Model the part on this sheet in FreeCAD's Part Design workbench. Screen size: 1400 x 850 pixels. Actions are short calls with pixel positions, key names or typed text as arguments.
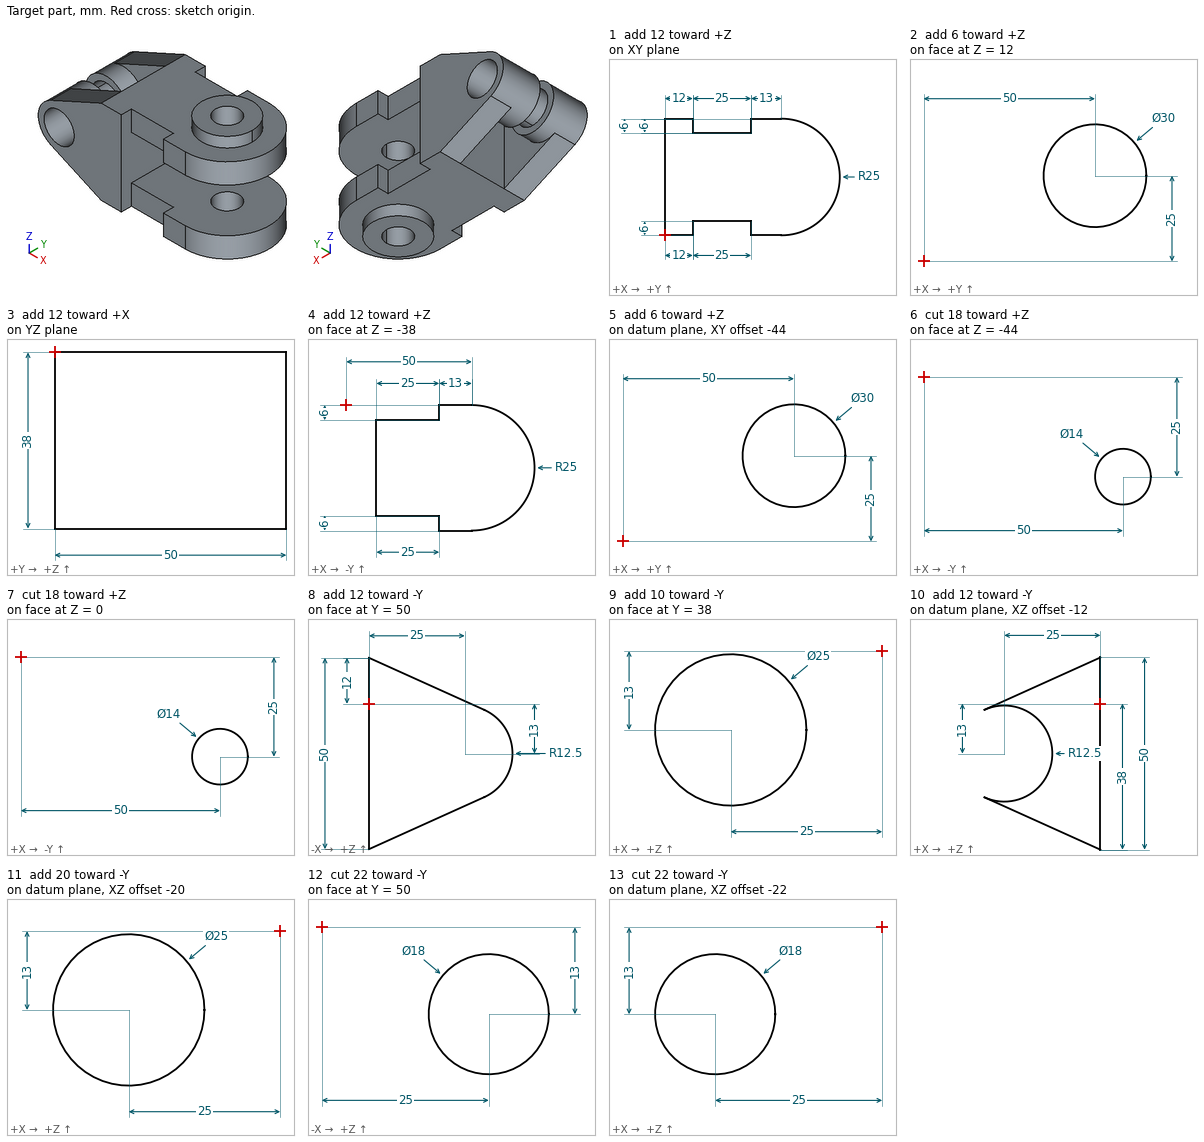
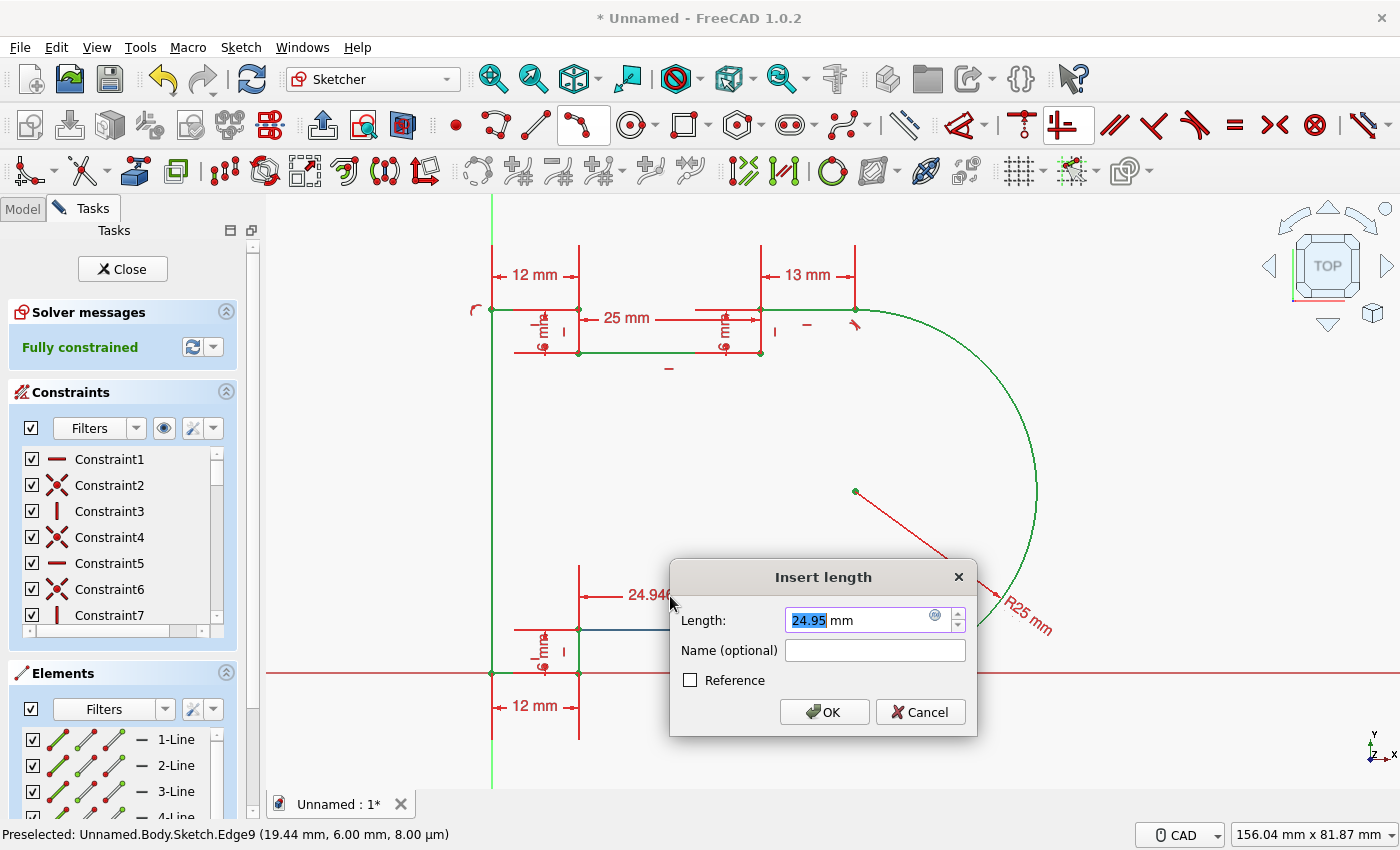
text(25)
key(Return)
key(Escape)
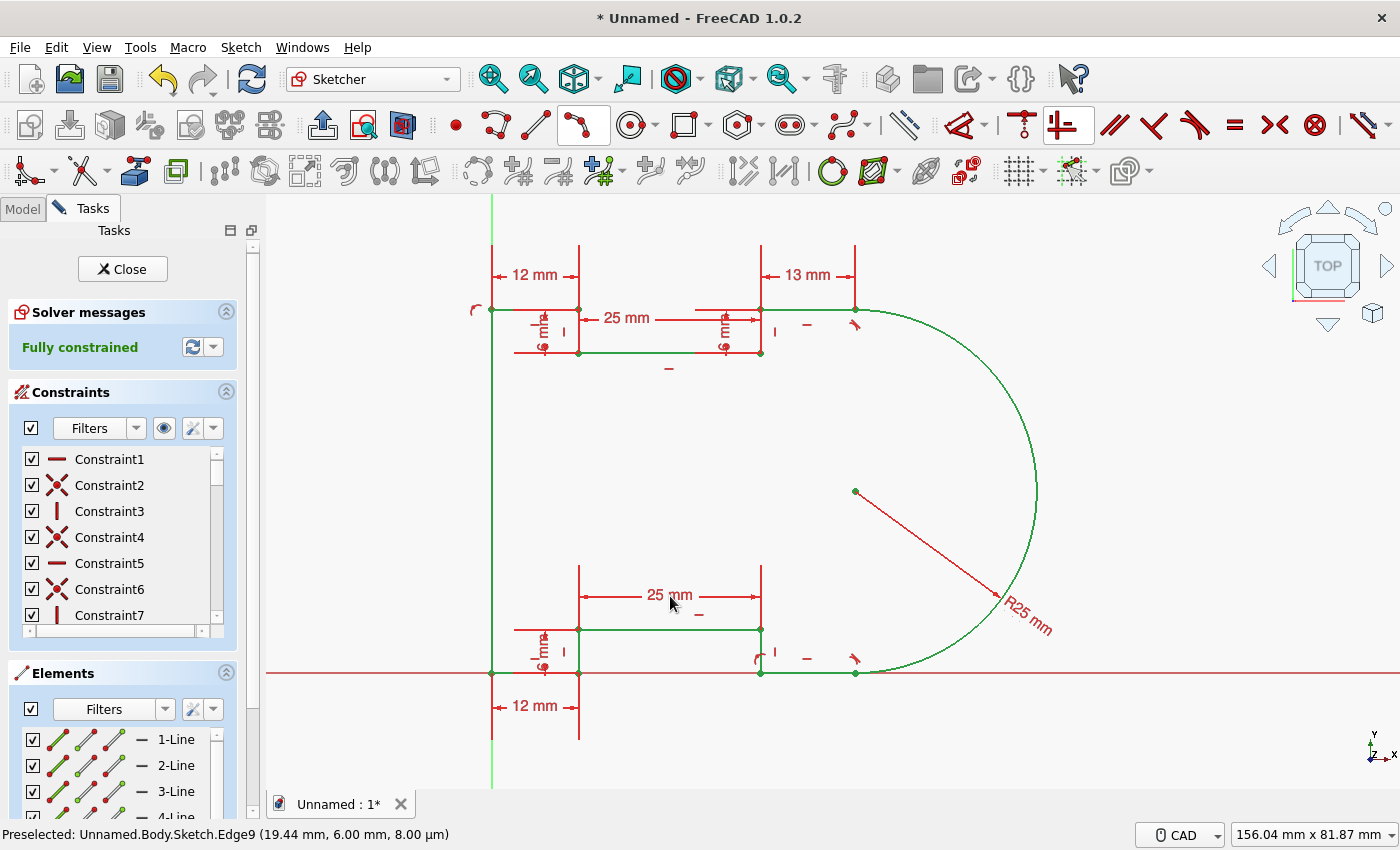
click(123, 269)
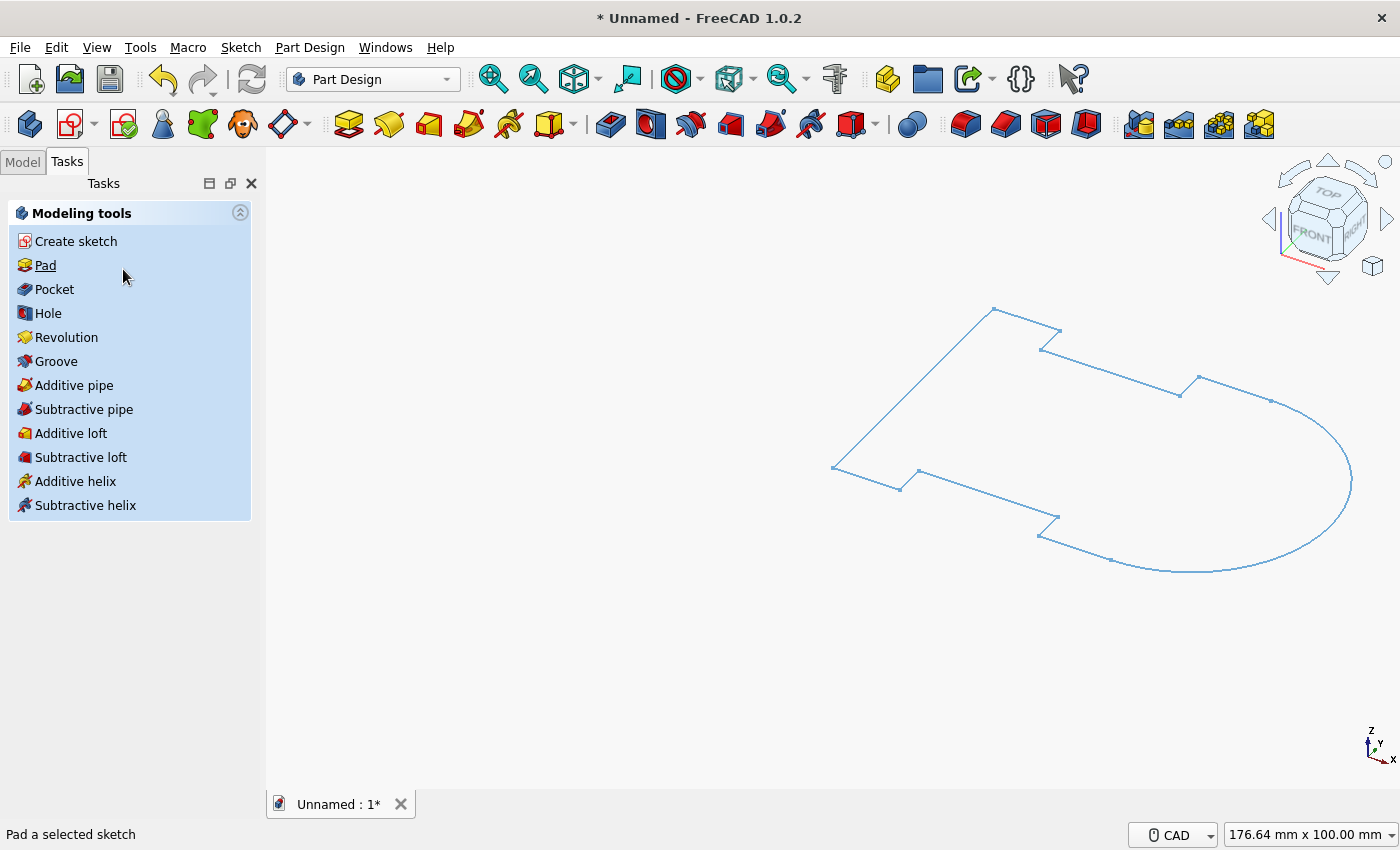
click(350, 124)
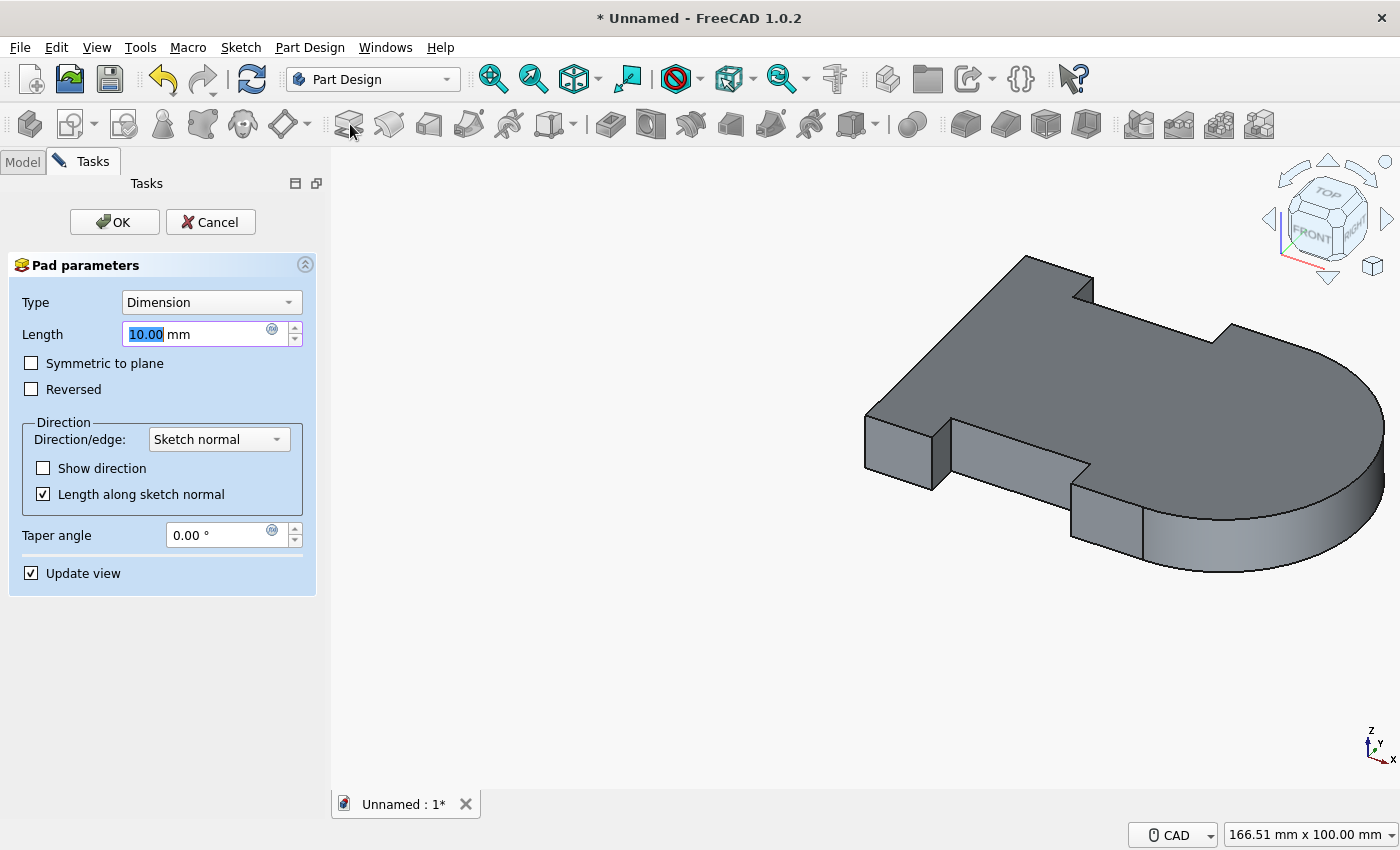
text(12)
key(Tab)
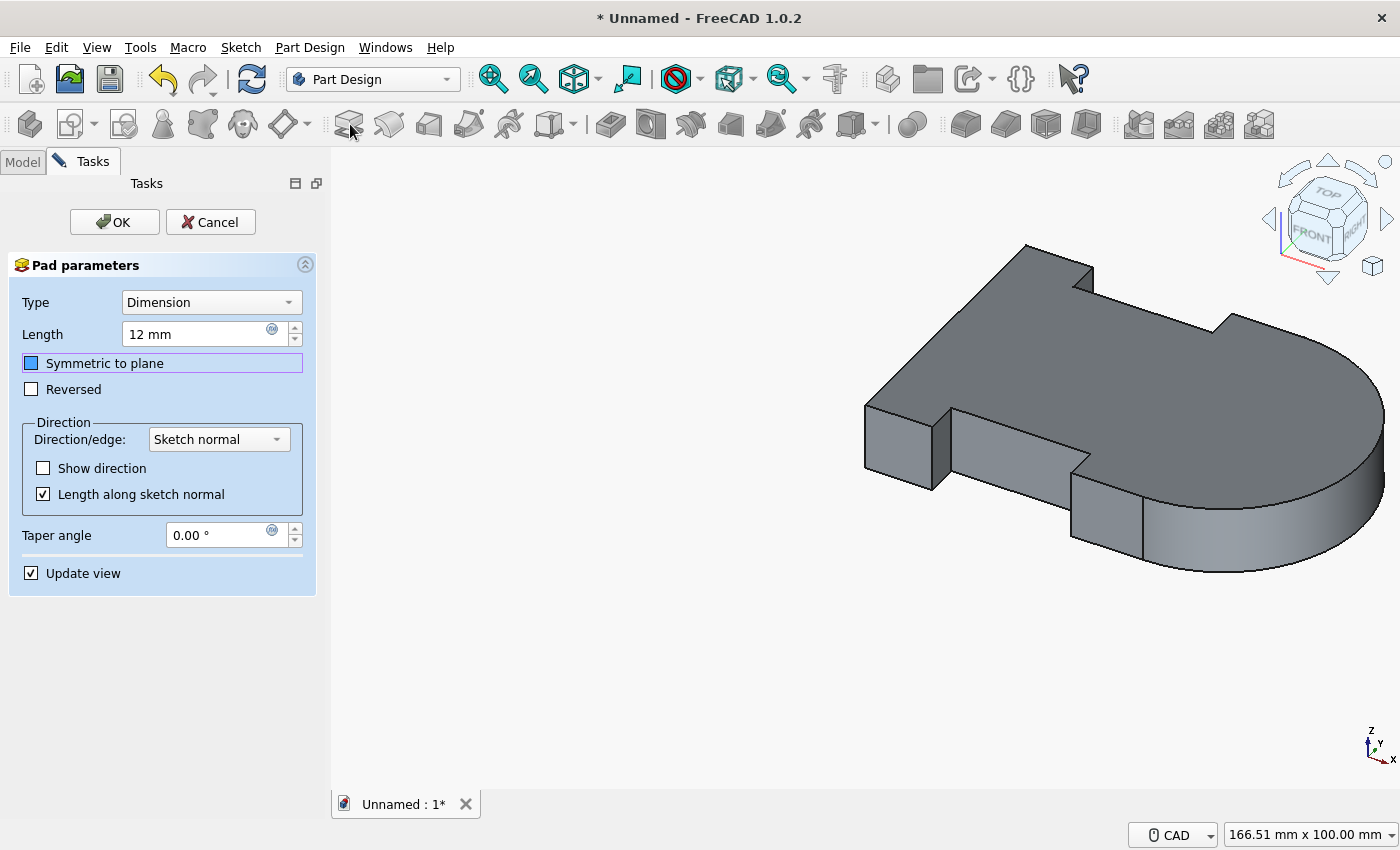
click(115, 222)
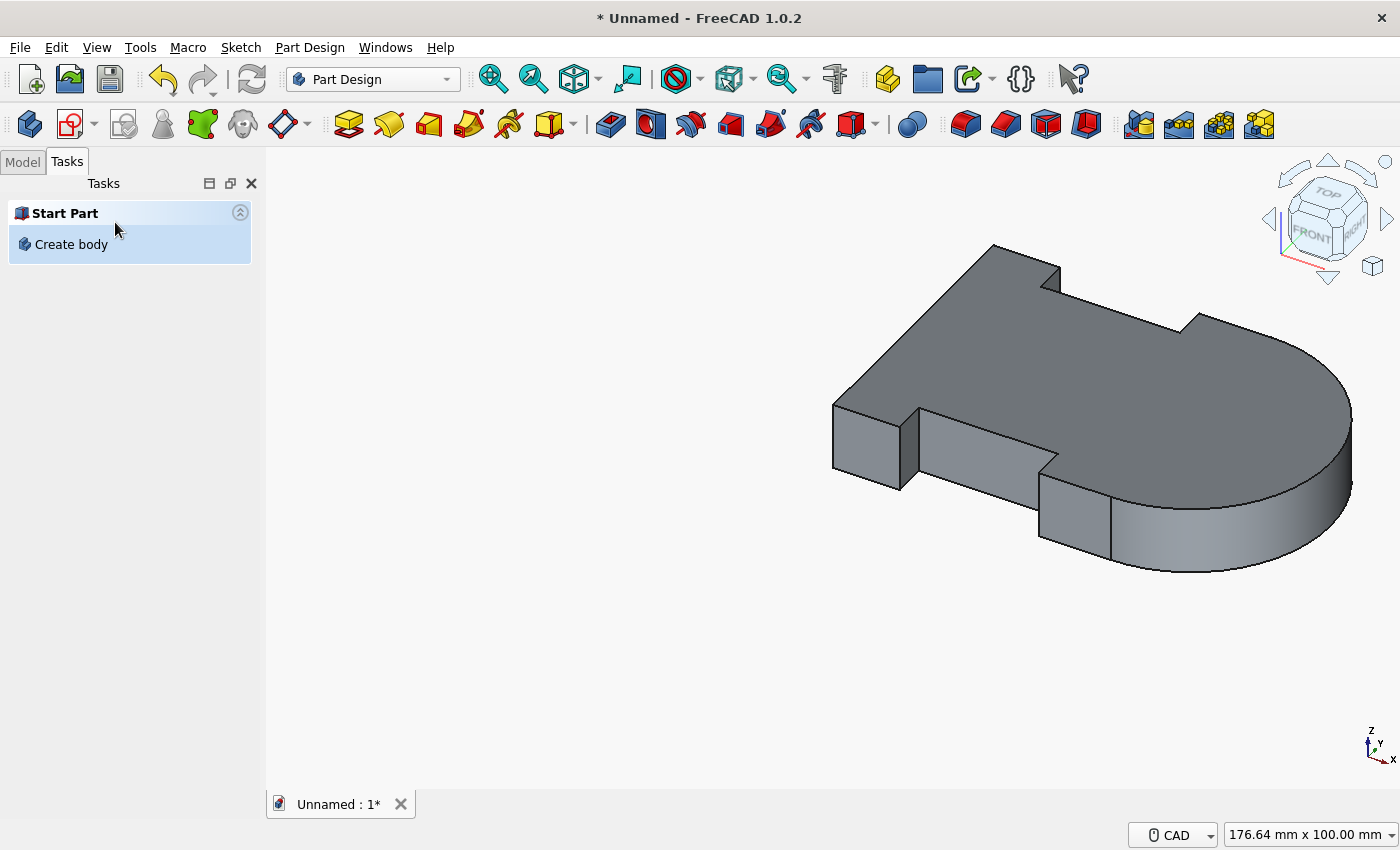
click(494, 80)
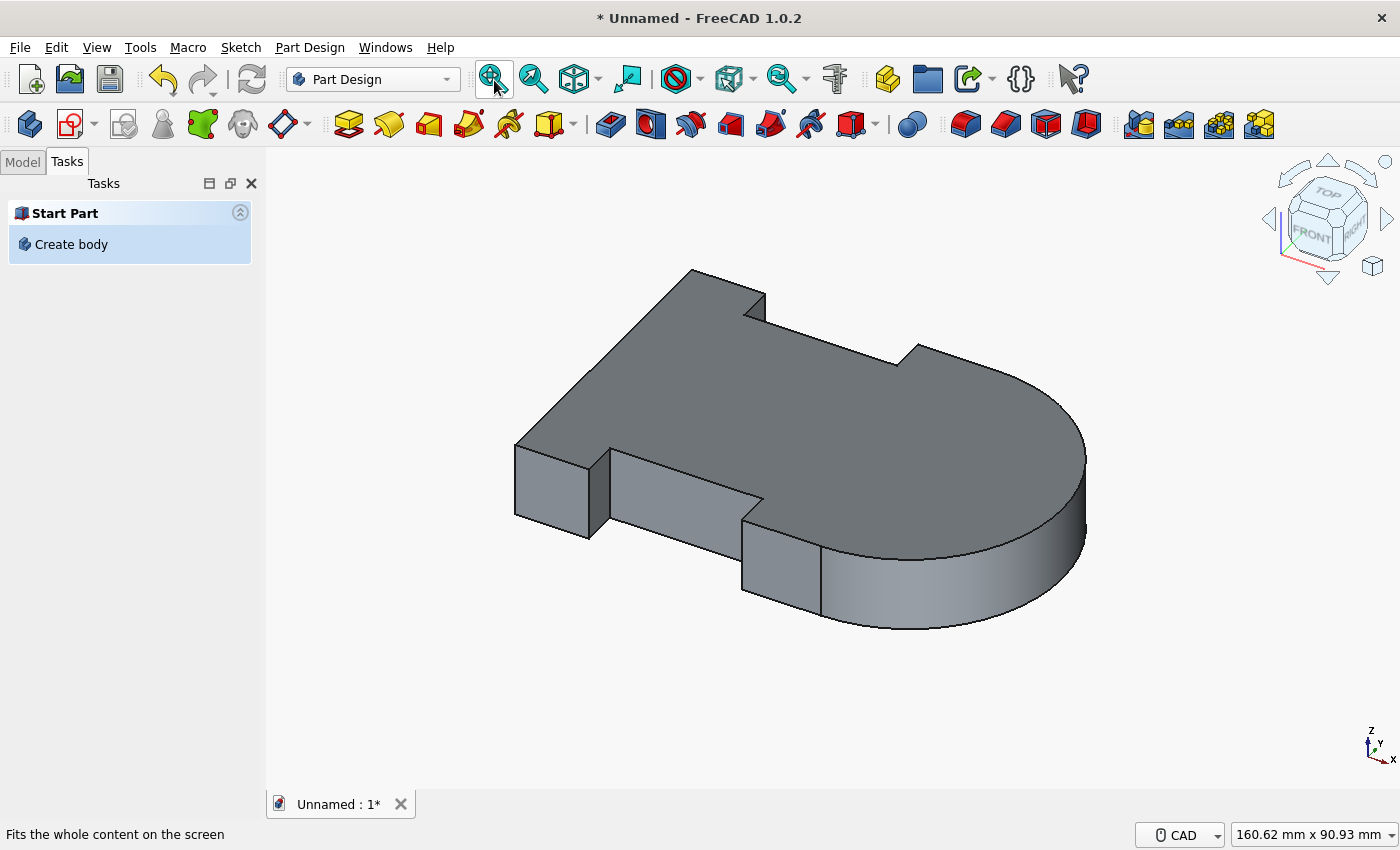
click(899, 454)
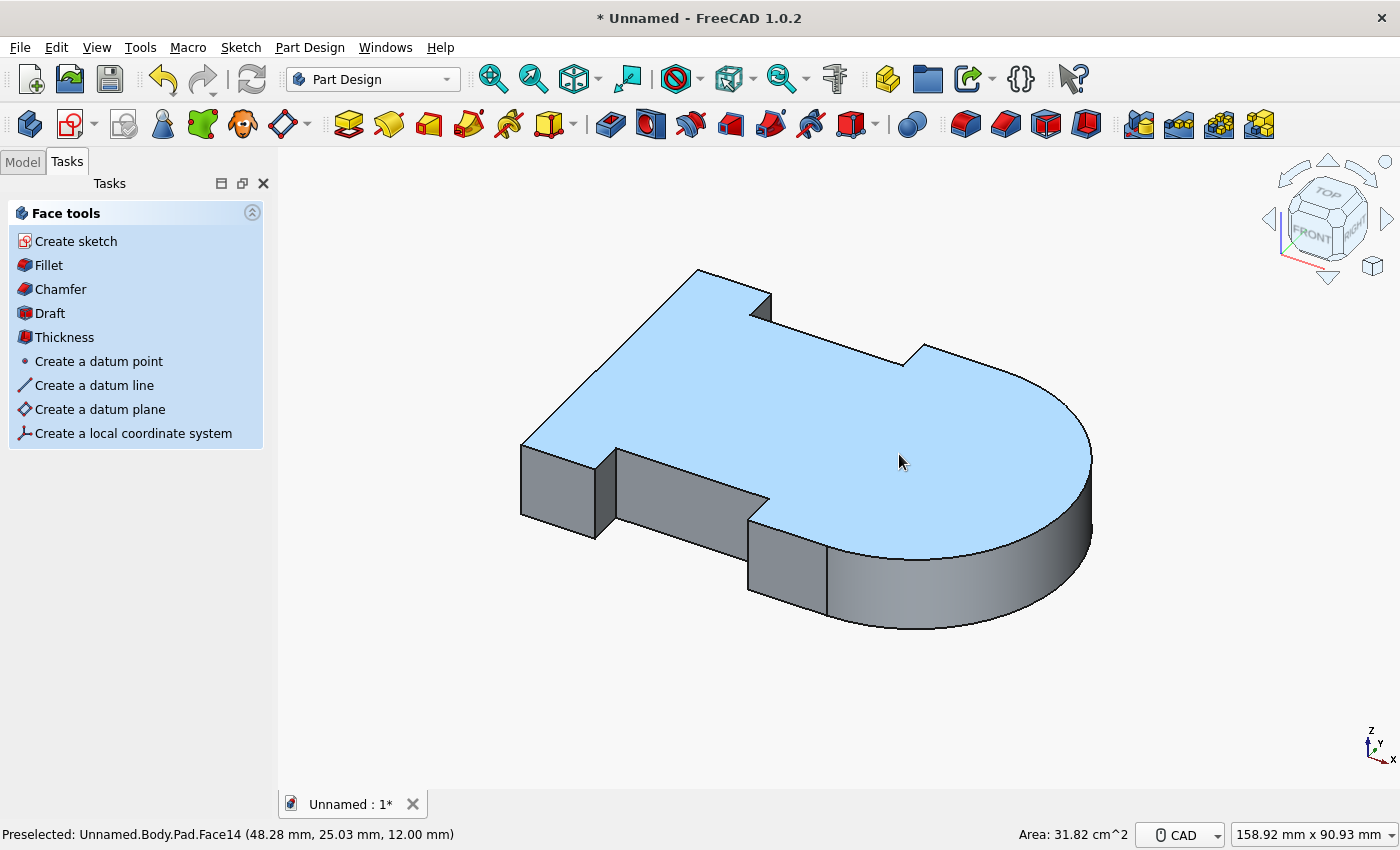
click(70, 124)